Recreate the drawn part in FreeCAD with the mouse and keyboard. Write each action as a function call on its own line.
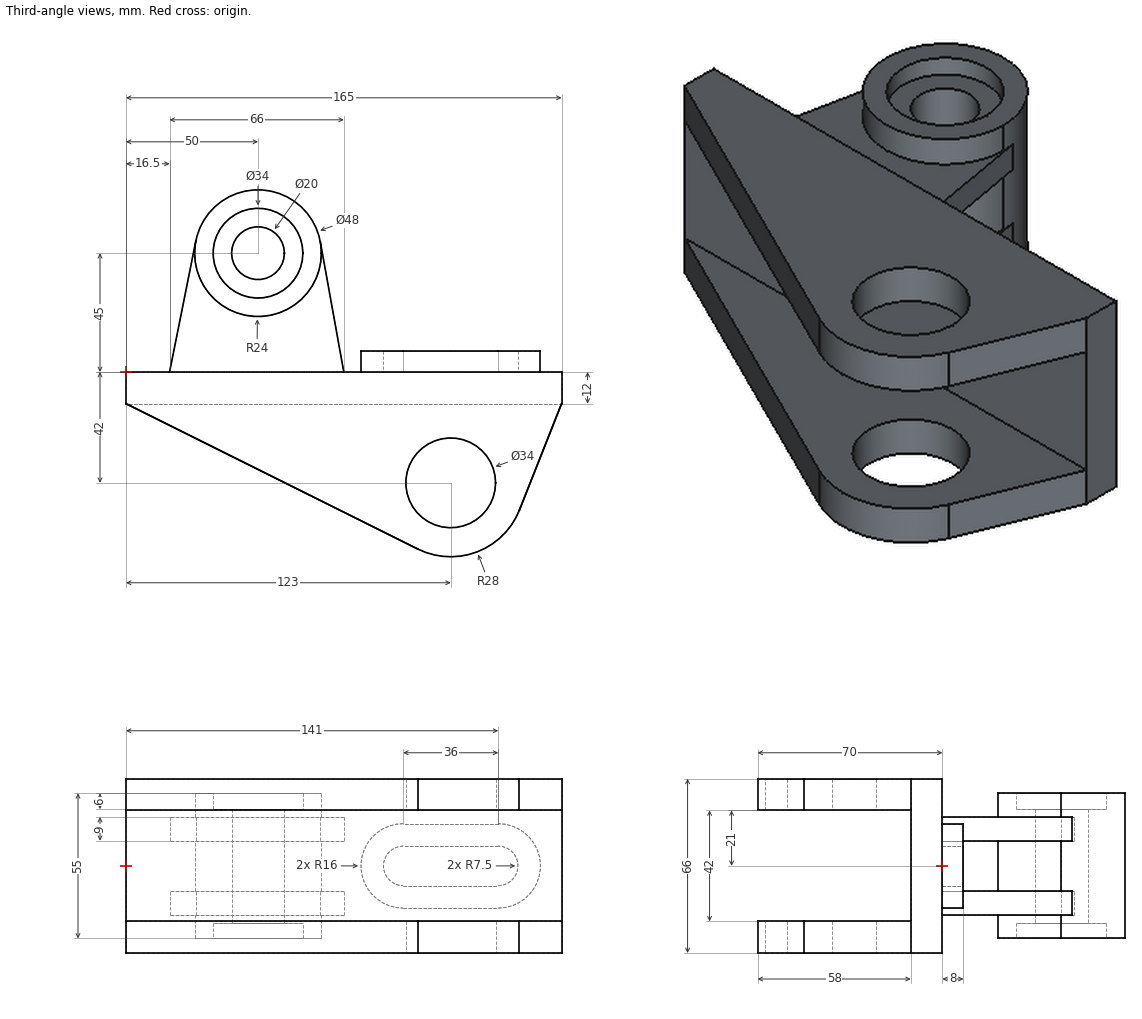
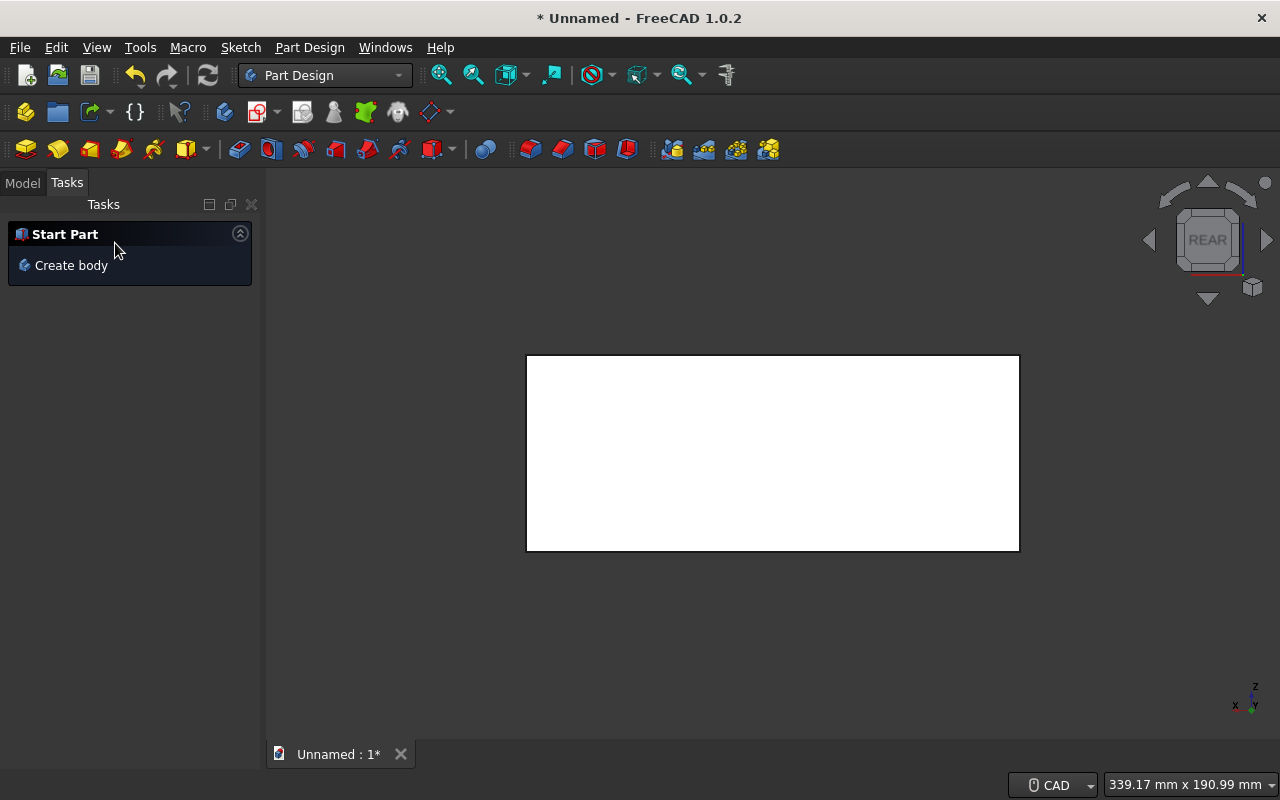
click(632, 452)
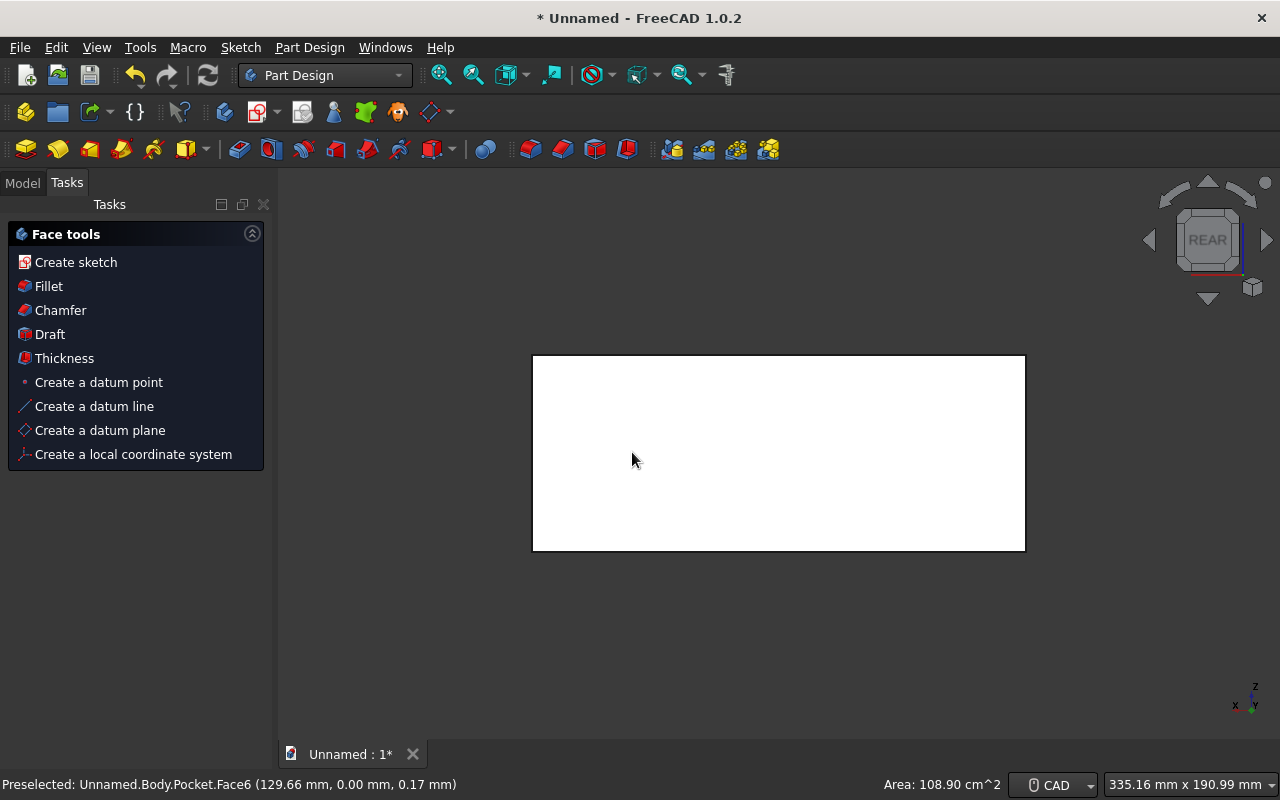
click(258, 112)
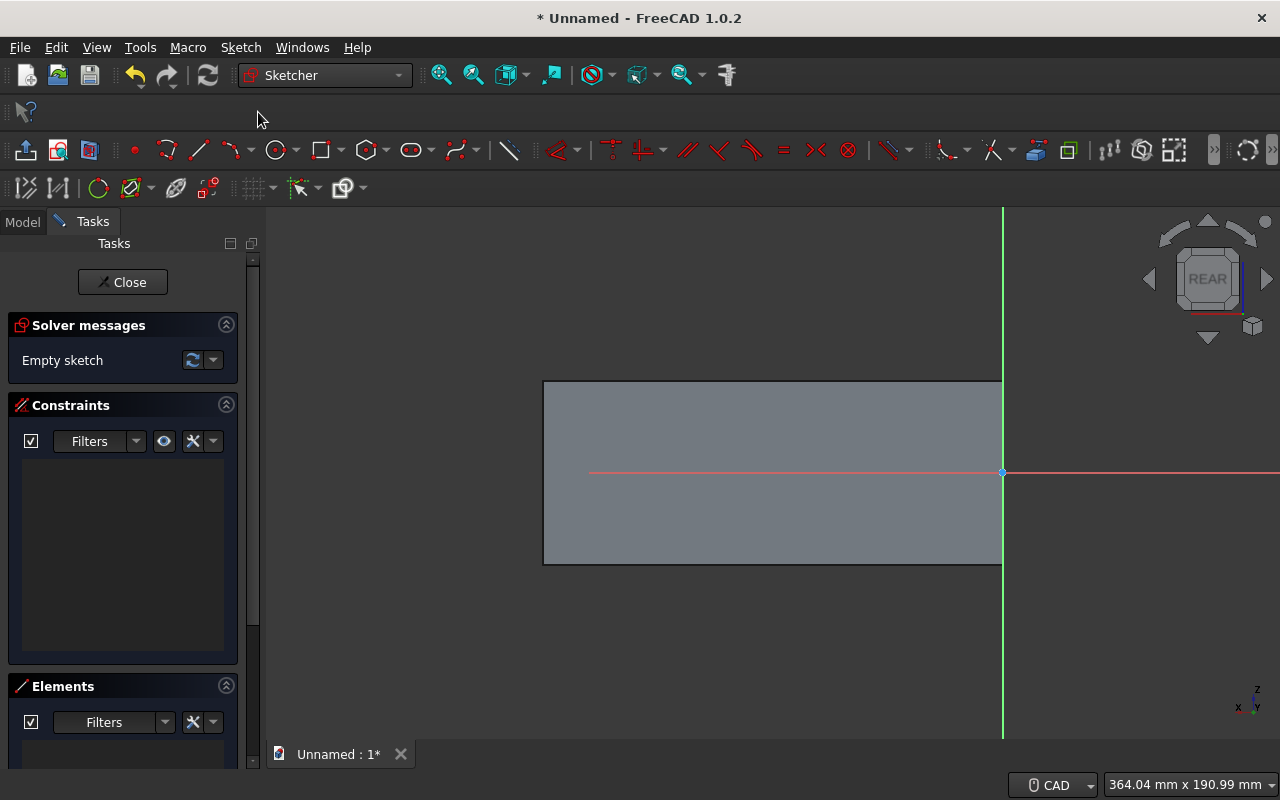
click(412, 150)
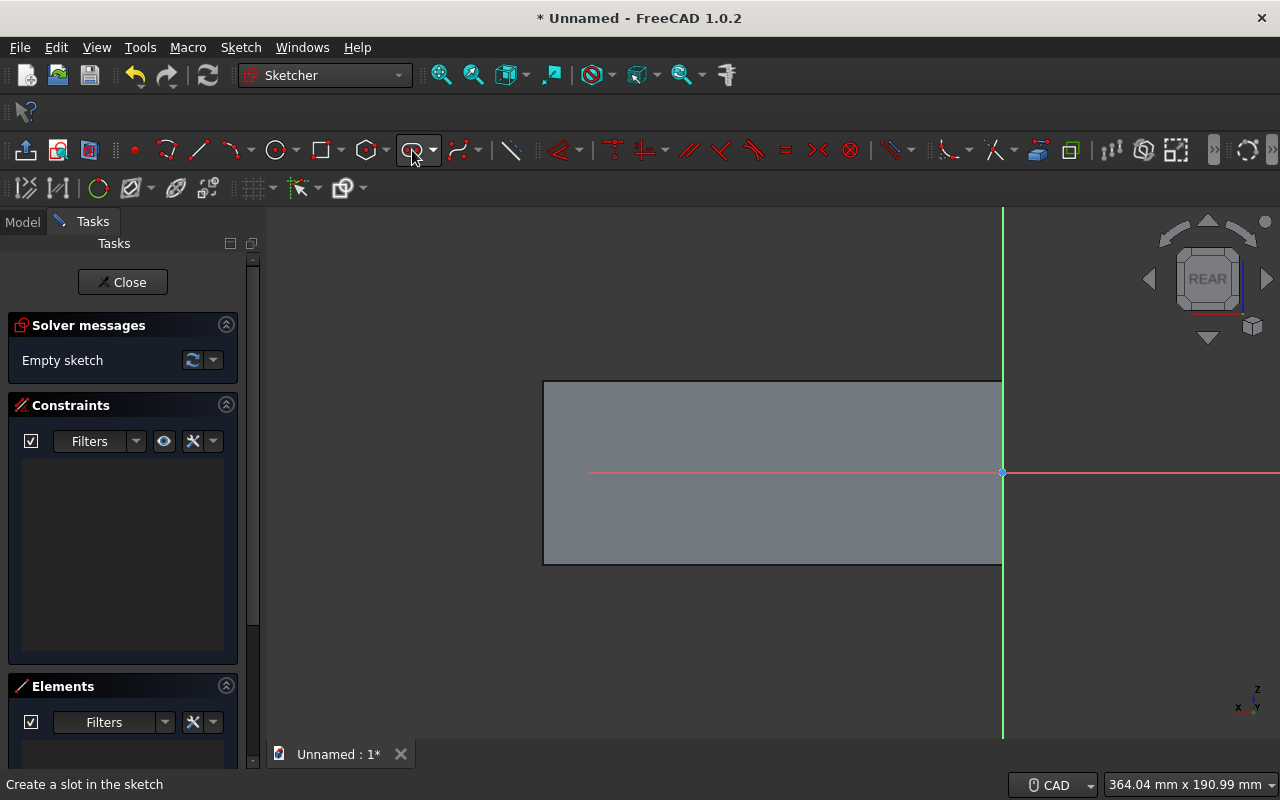
click(610, 473)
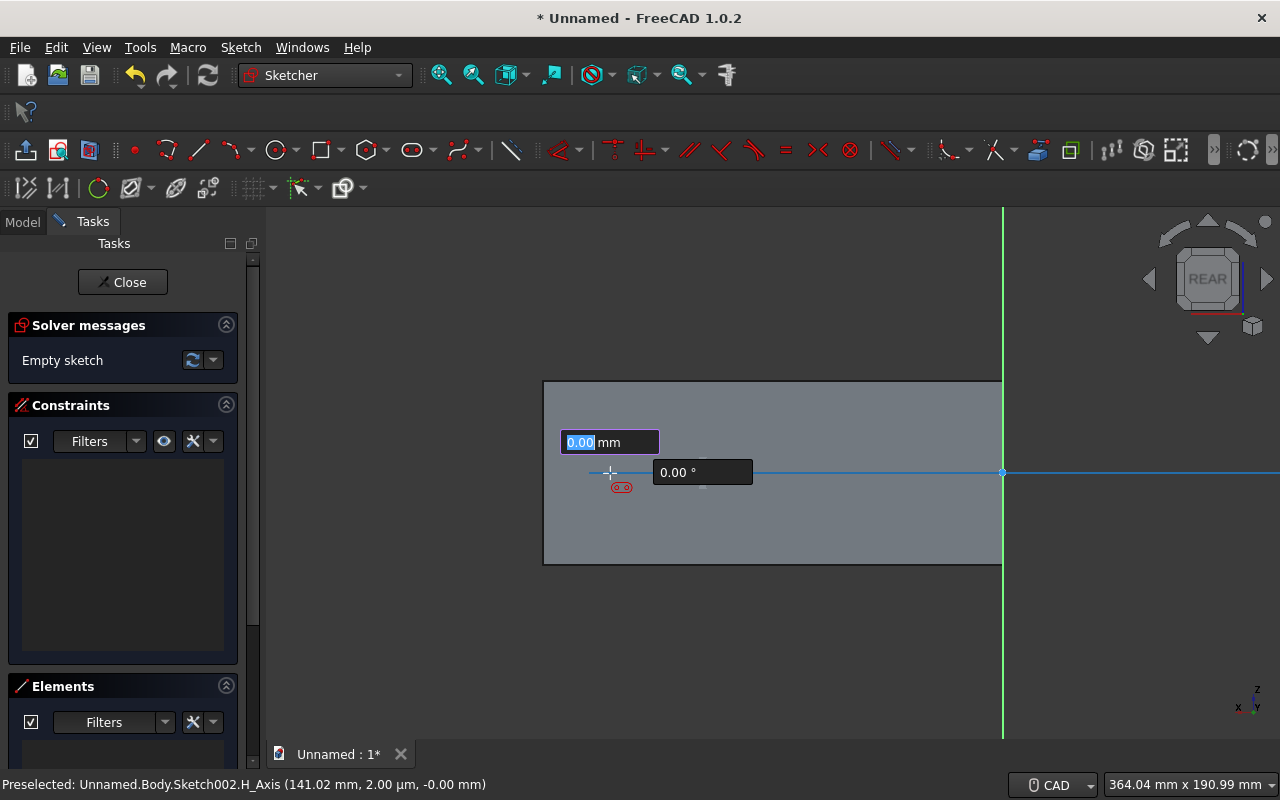
click(710, 464)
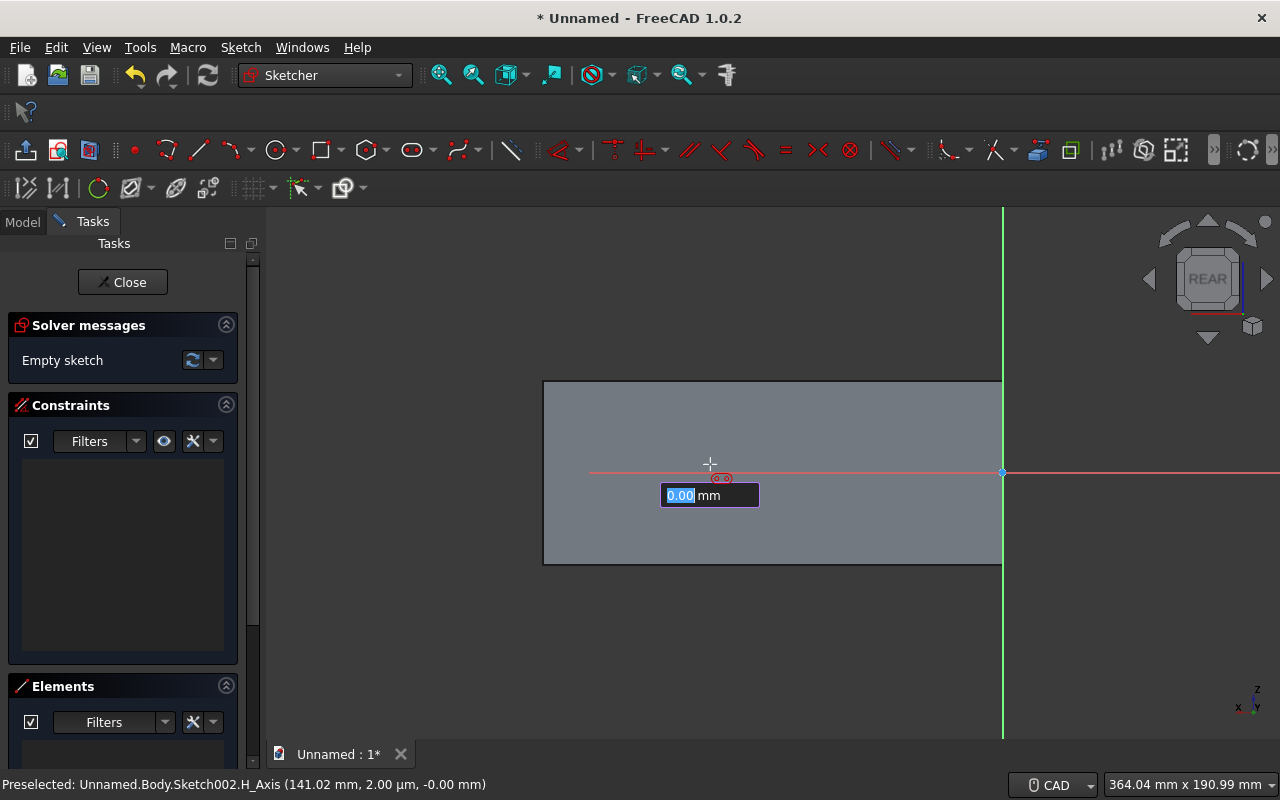
click(660, 518)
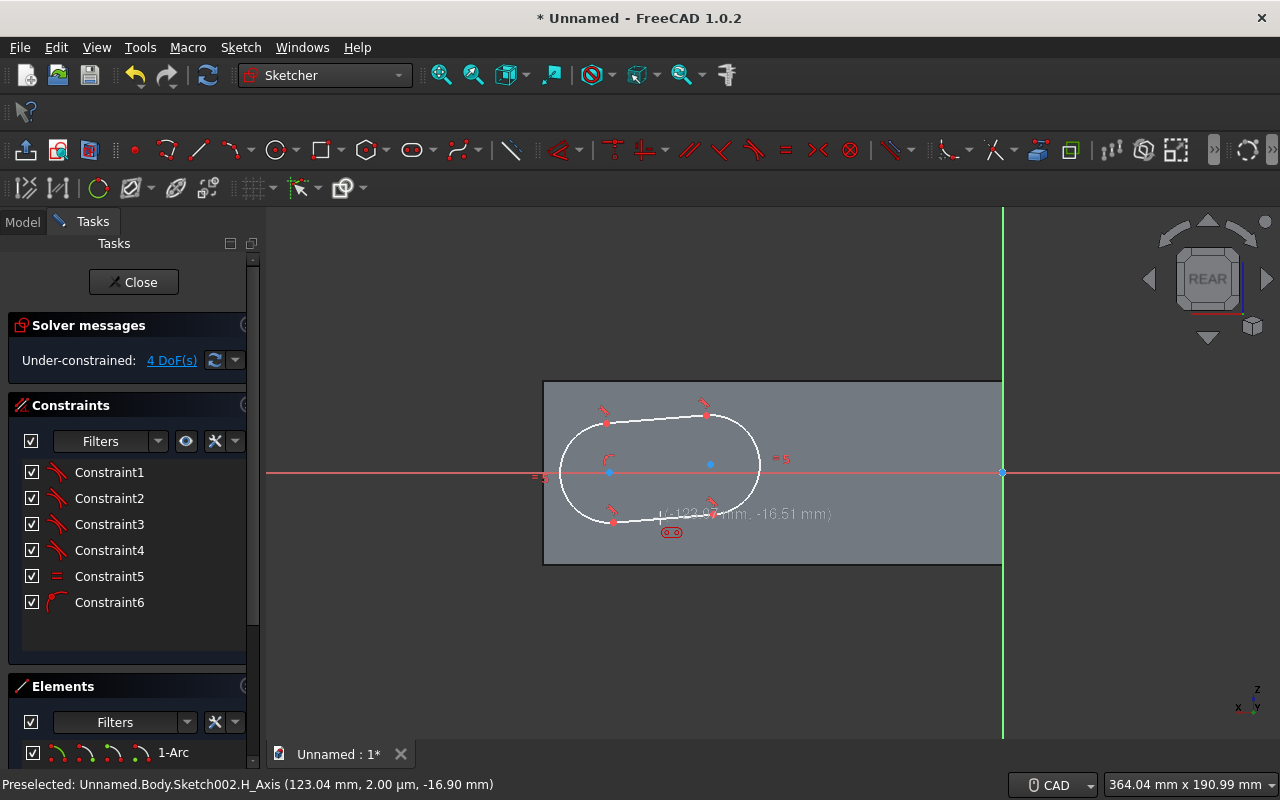
click(610, 473)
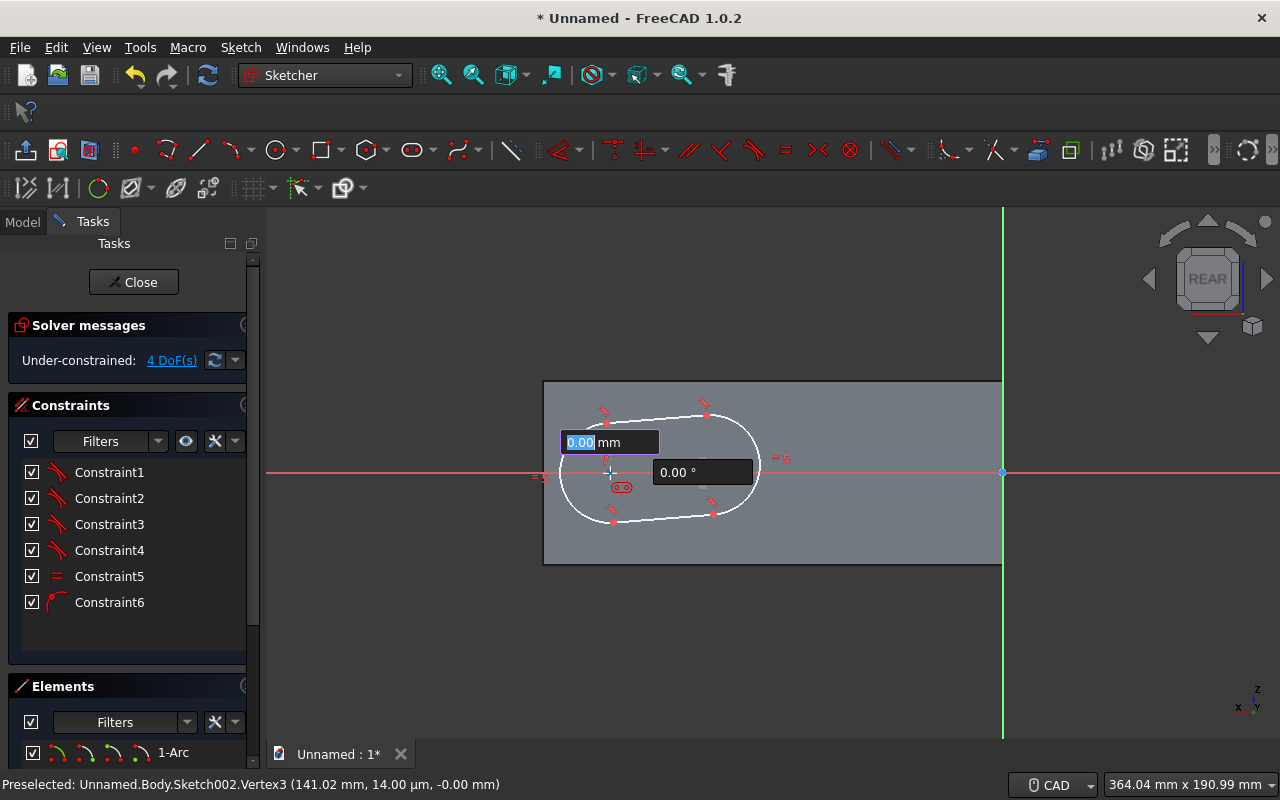
click(710, 465)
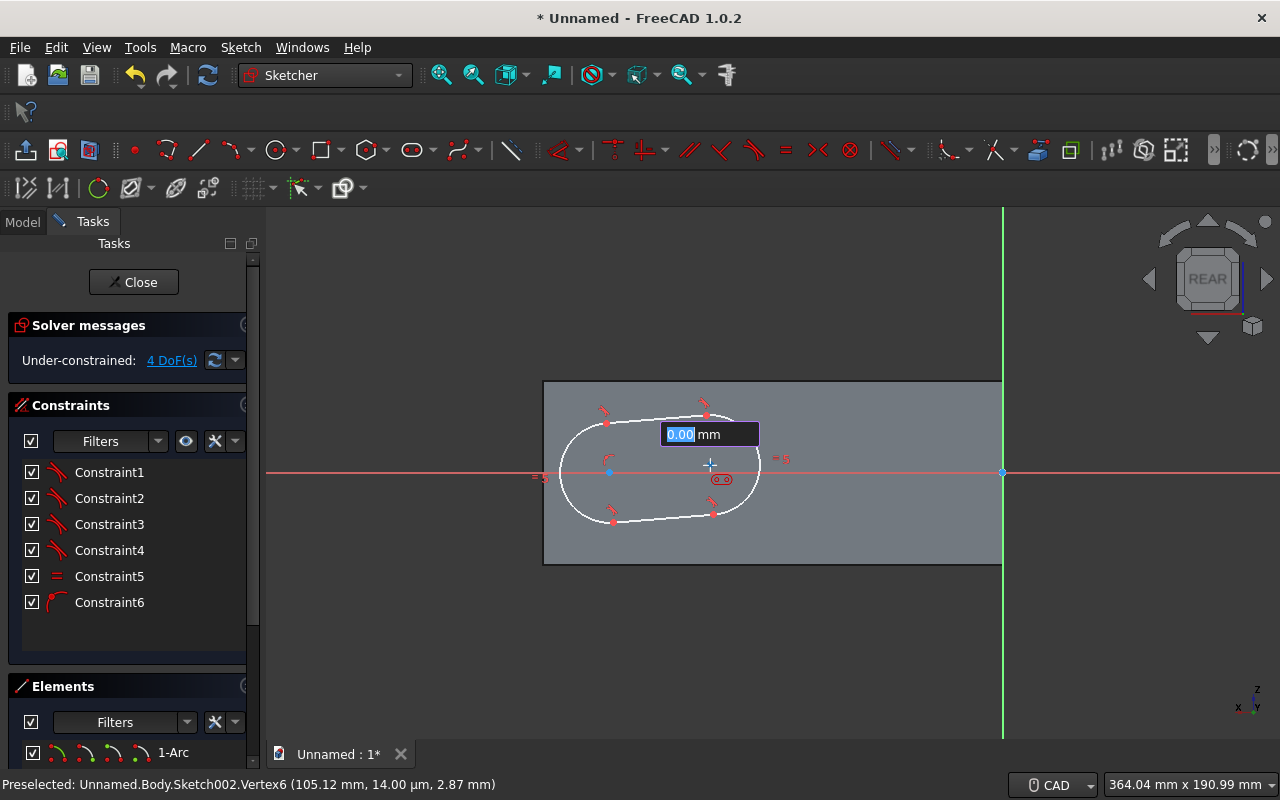
click(660, 494)
key(Escape)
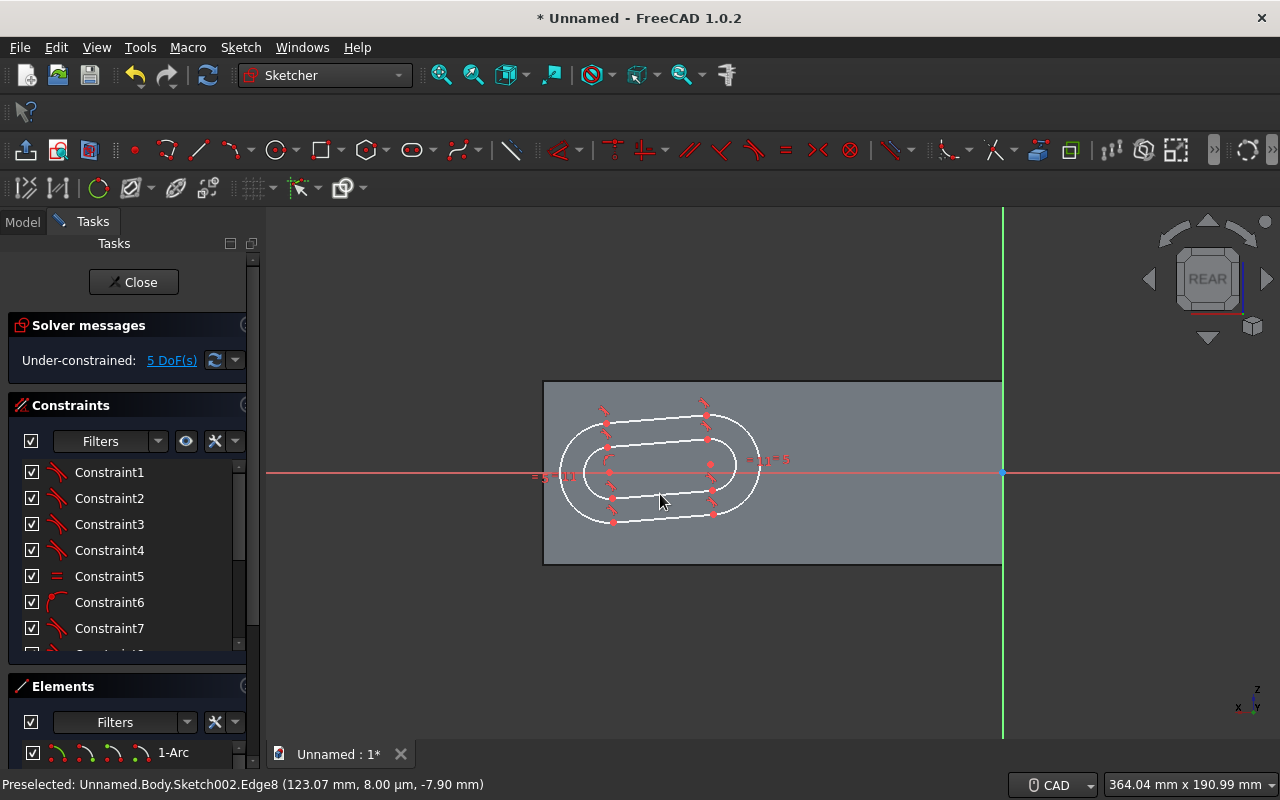
click(636, 421)